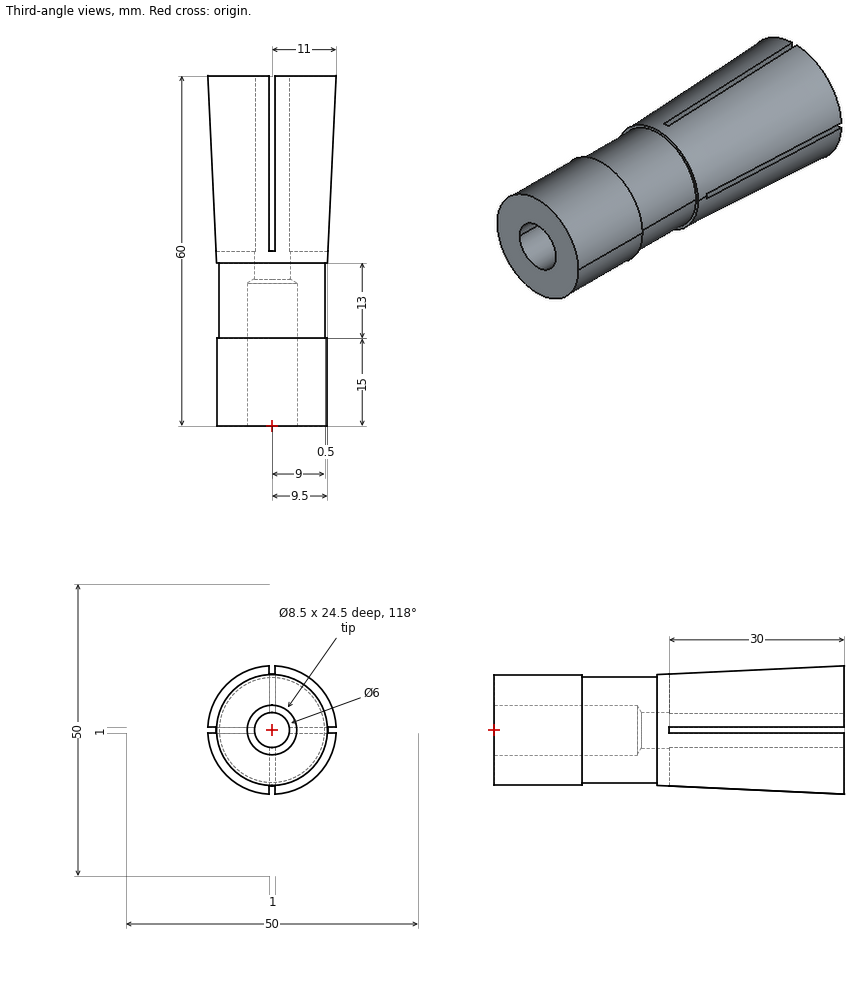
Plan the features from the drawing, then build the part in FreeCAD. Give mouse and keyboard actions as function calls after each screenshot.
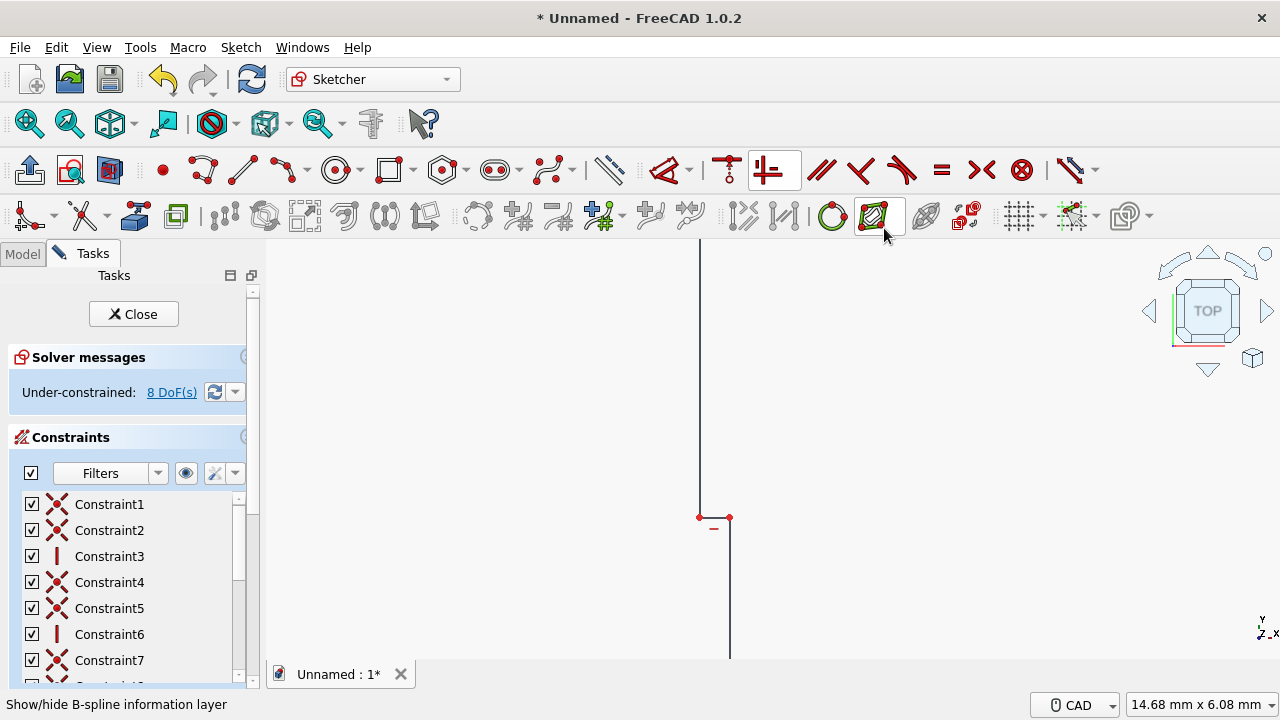
scroll(720, 513, down, 14)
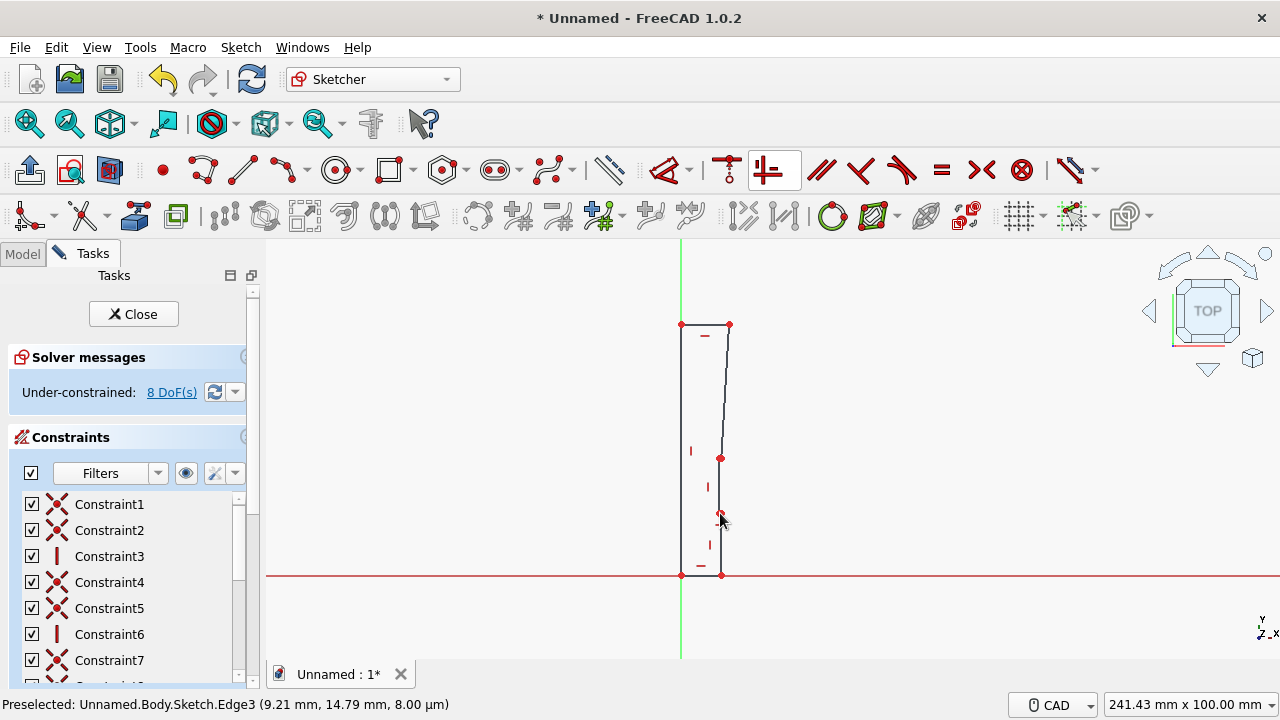
scroll(720, 459, up, 14)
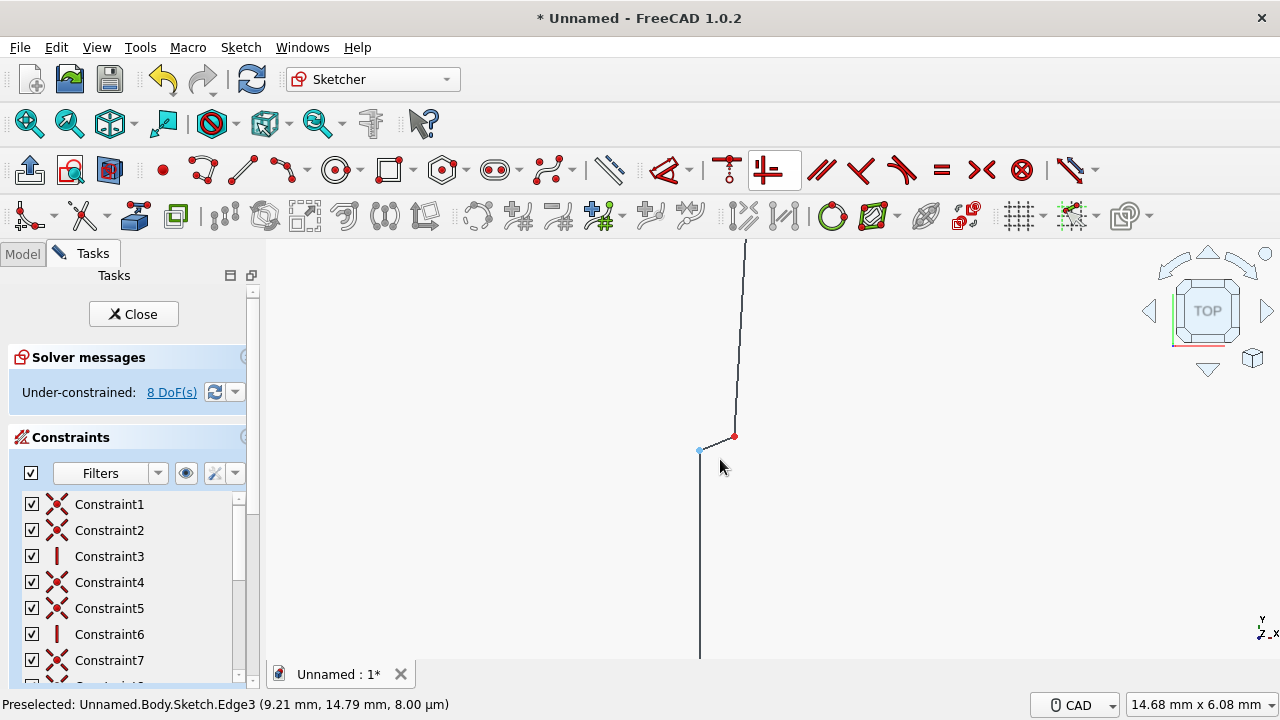
click(710, 447)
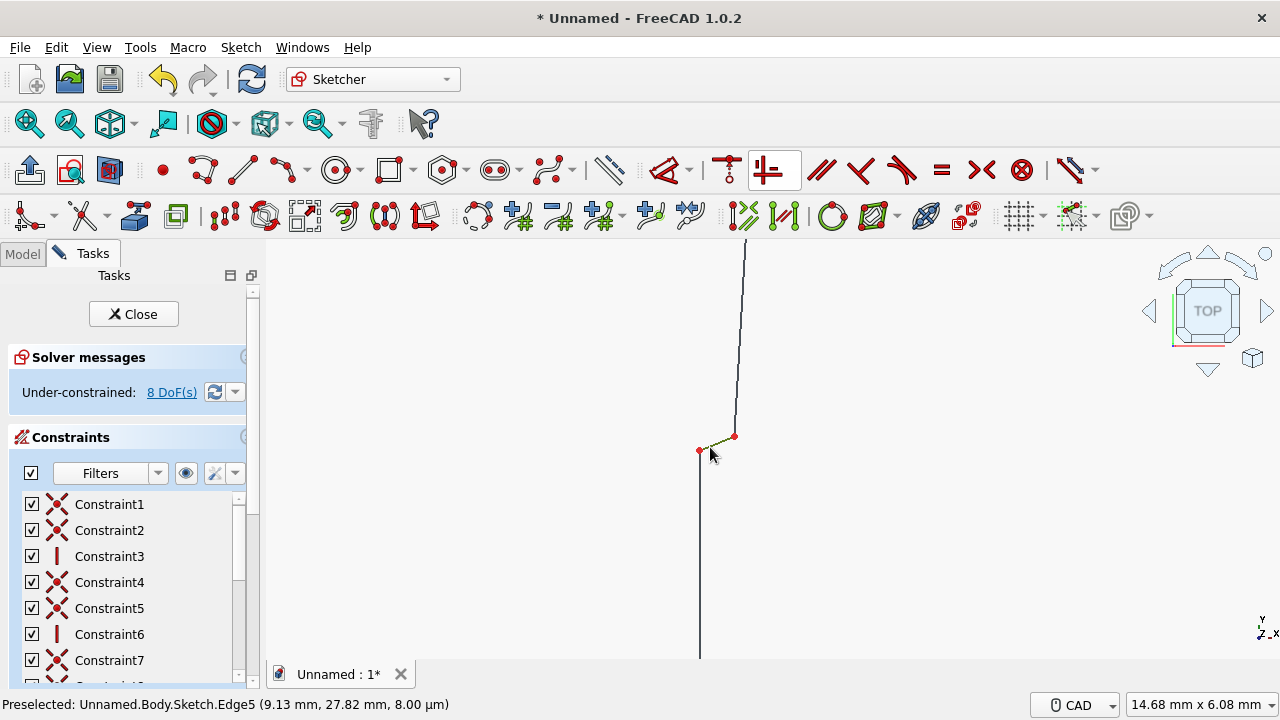
click(796, 170)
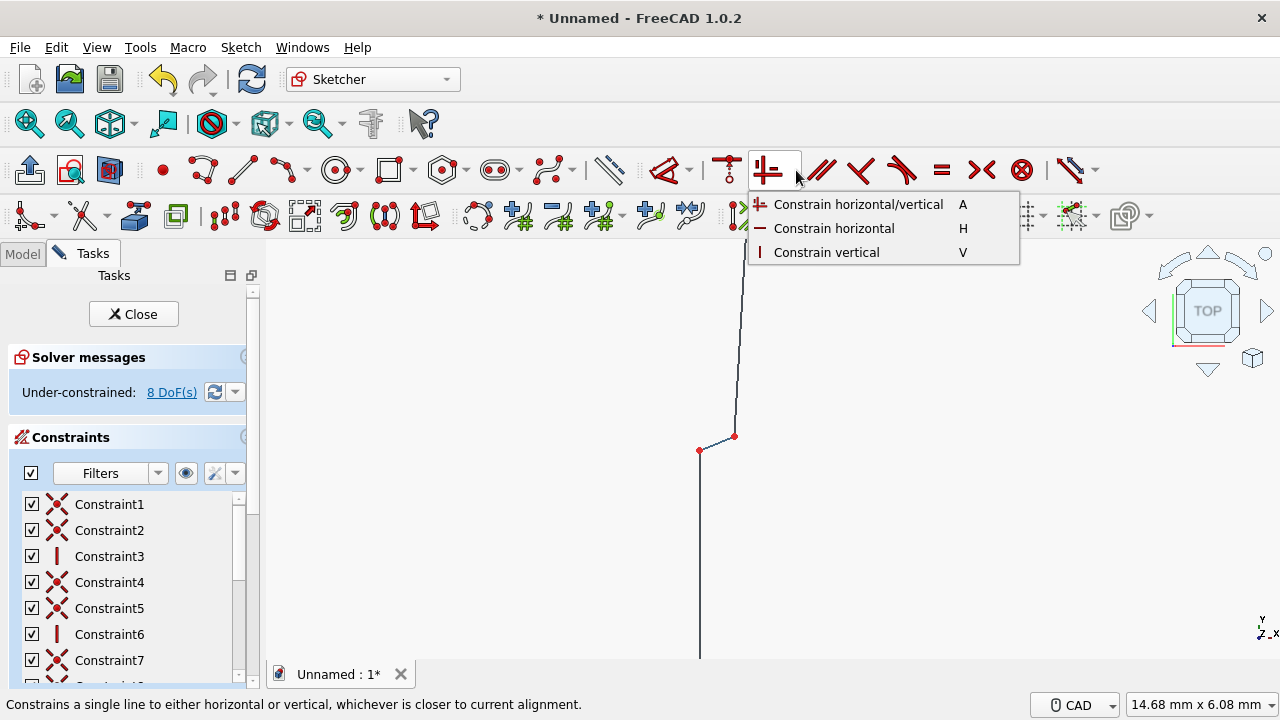
click(884, 228)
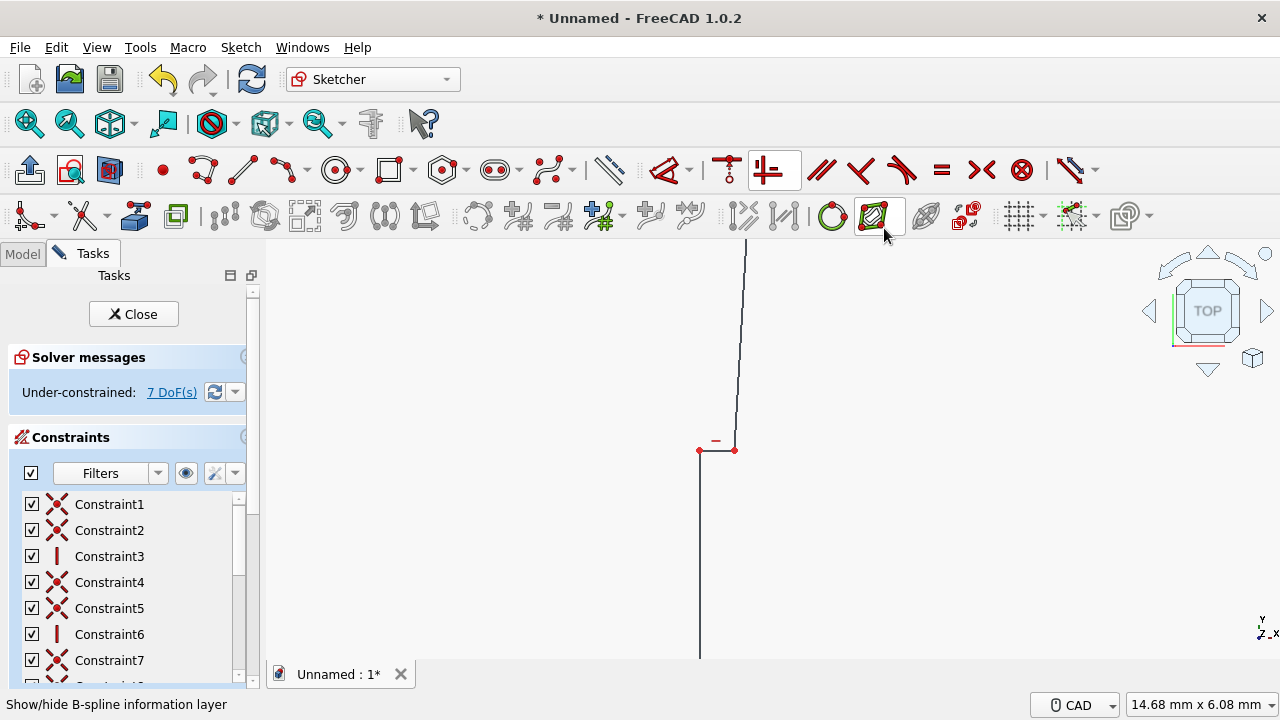
scroll(720, 459, down, 14)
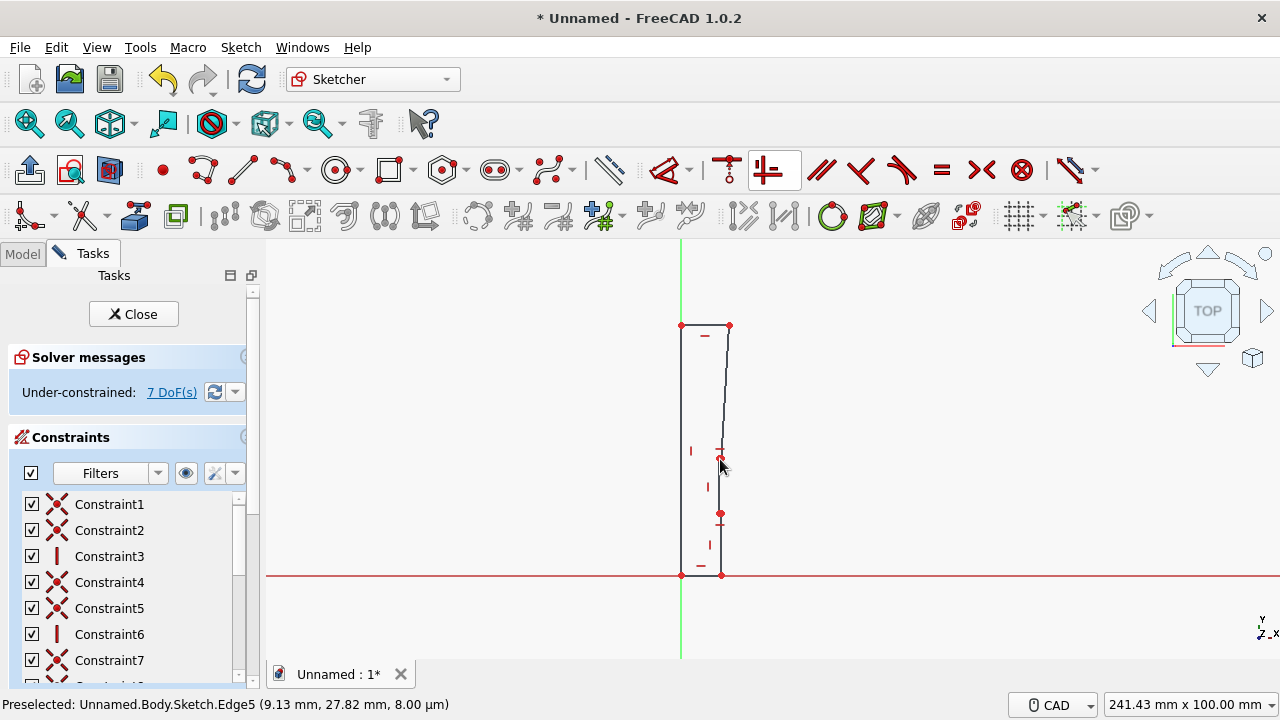
click(721, 557)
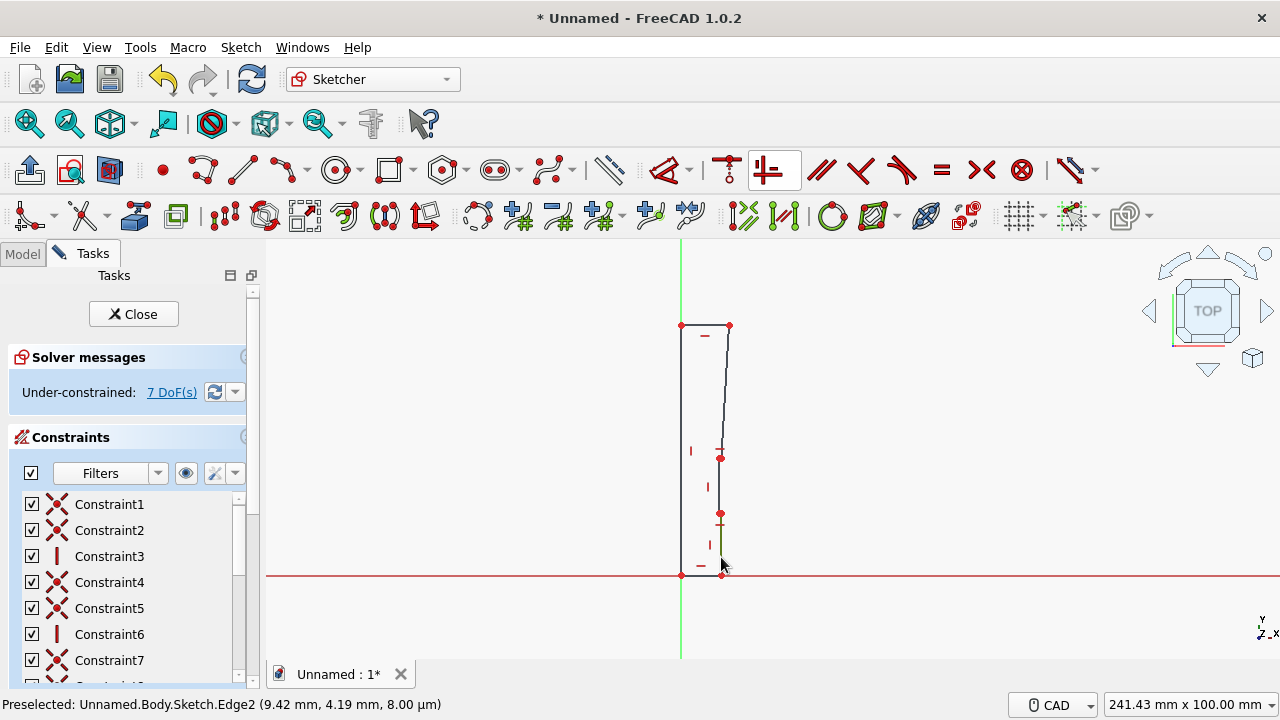
key(i)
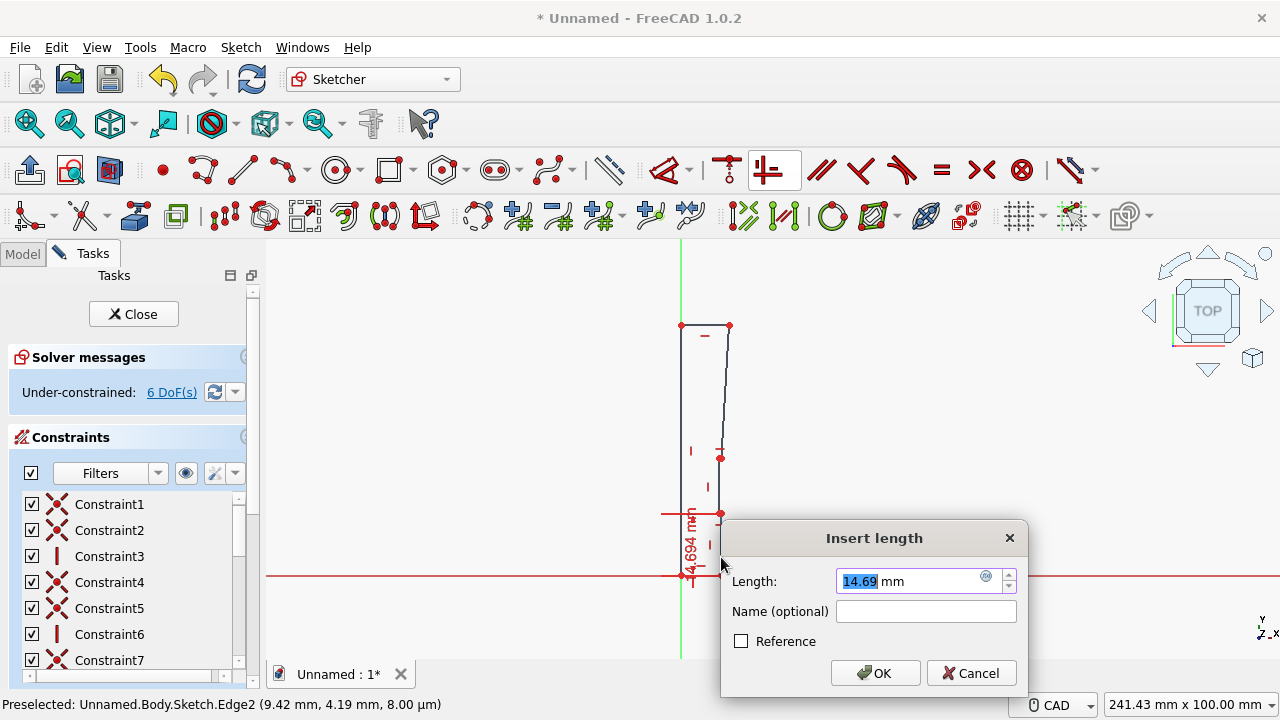
text(15)
key(Return)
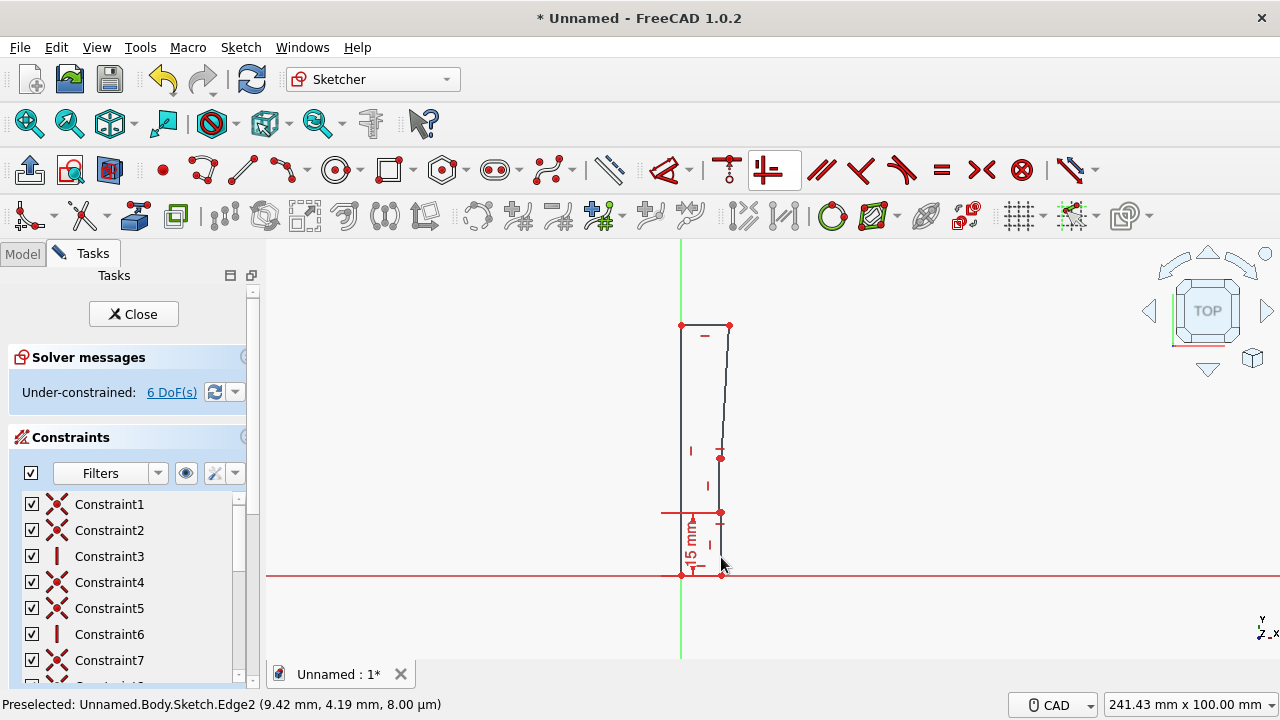
click(719, 497)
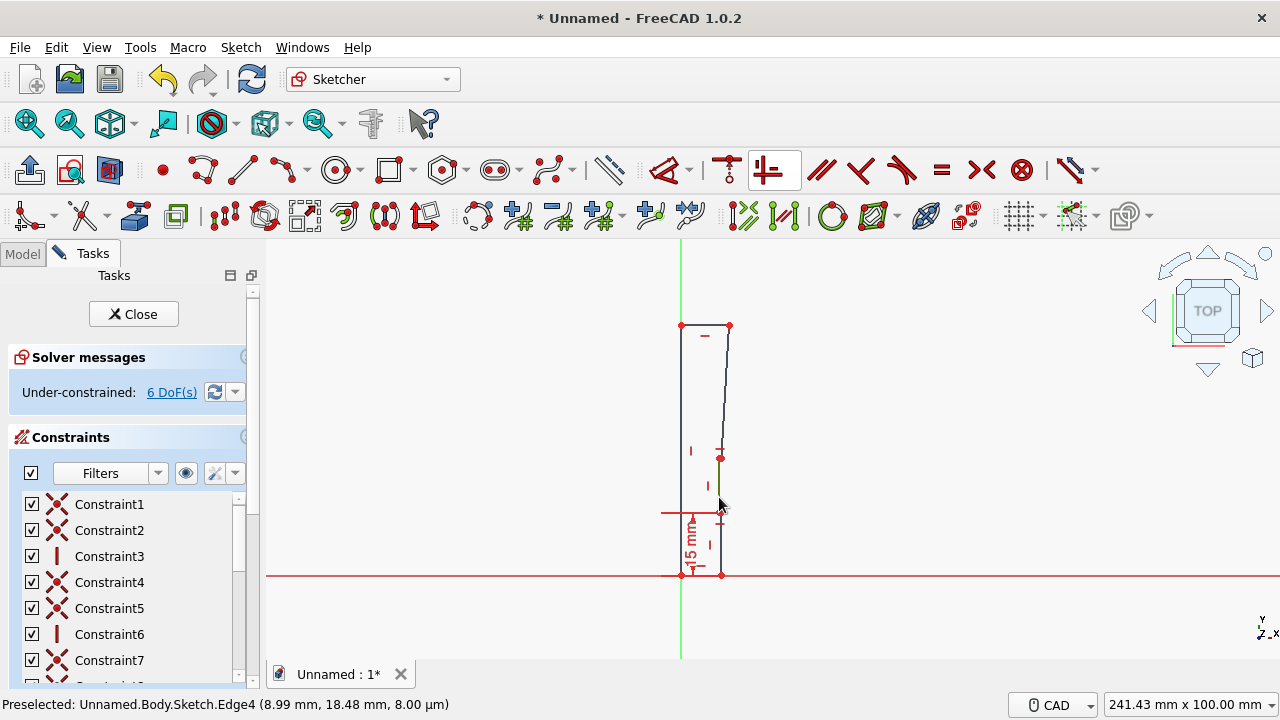
key(i)